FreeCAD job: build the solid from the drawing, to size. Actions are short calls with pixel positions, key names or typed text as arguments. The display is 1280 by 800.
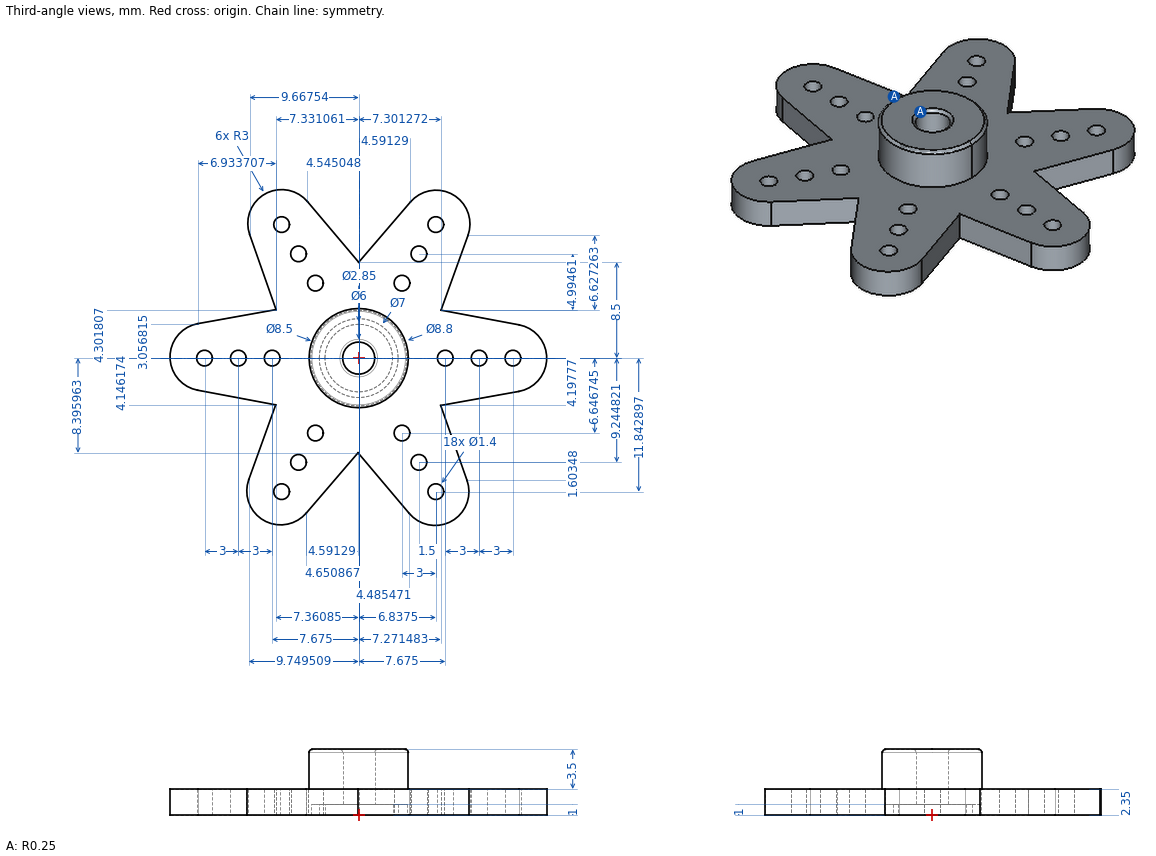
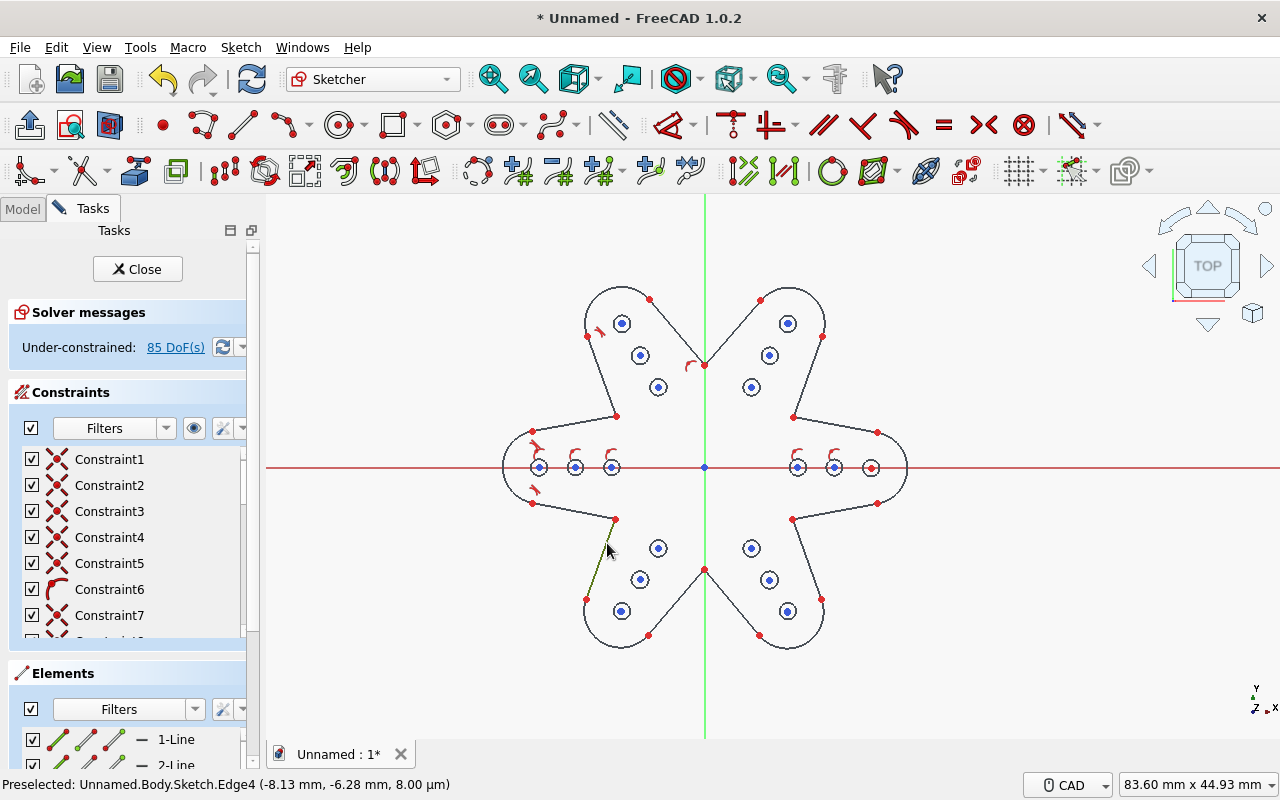
click(589, 628)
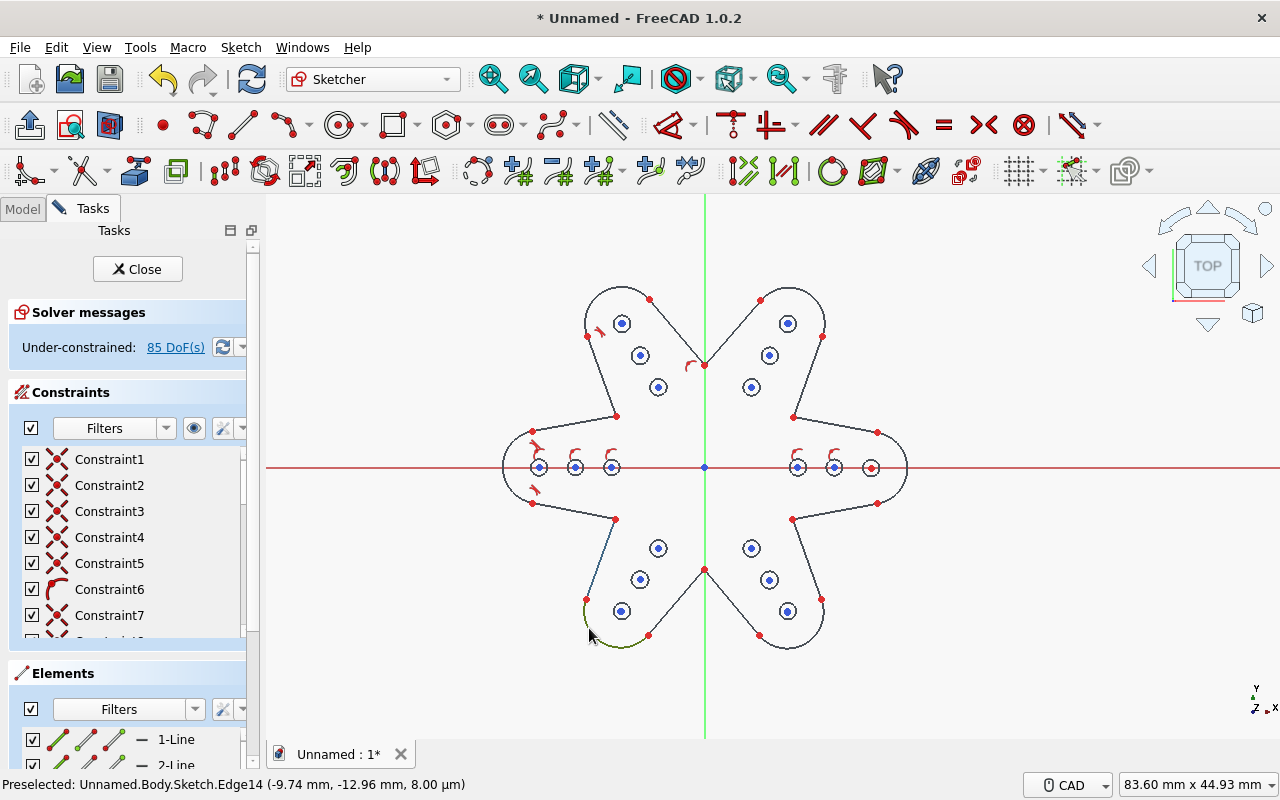
click(904, 126)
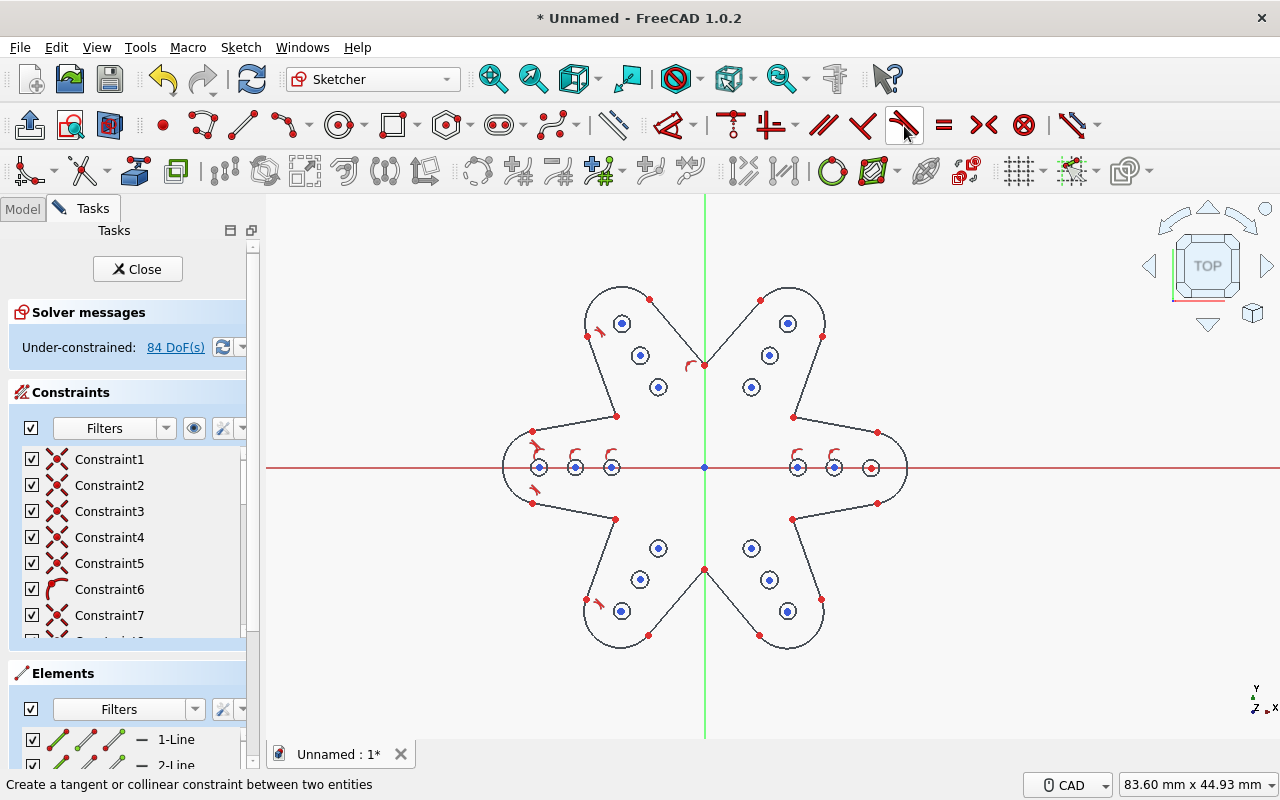
click(665, 615)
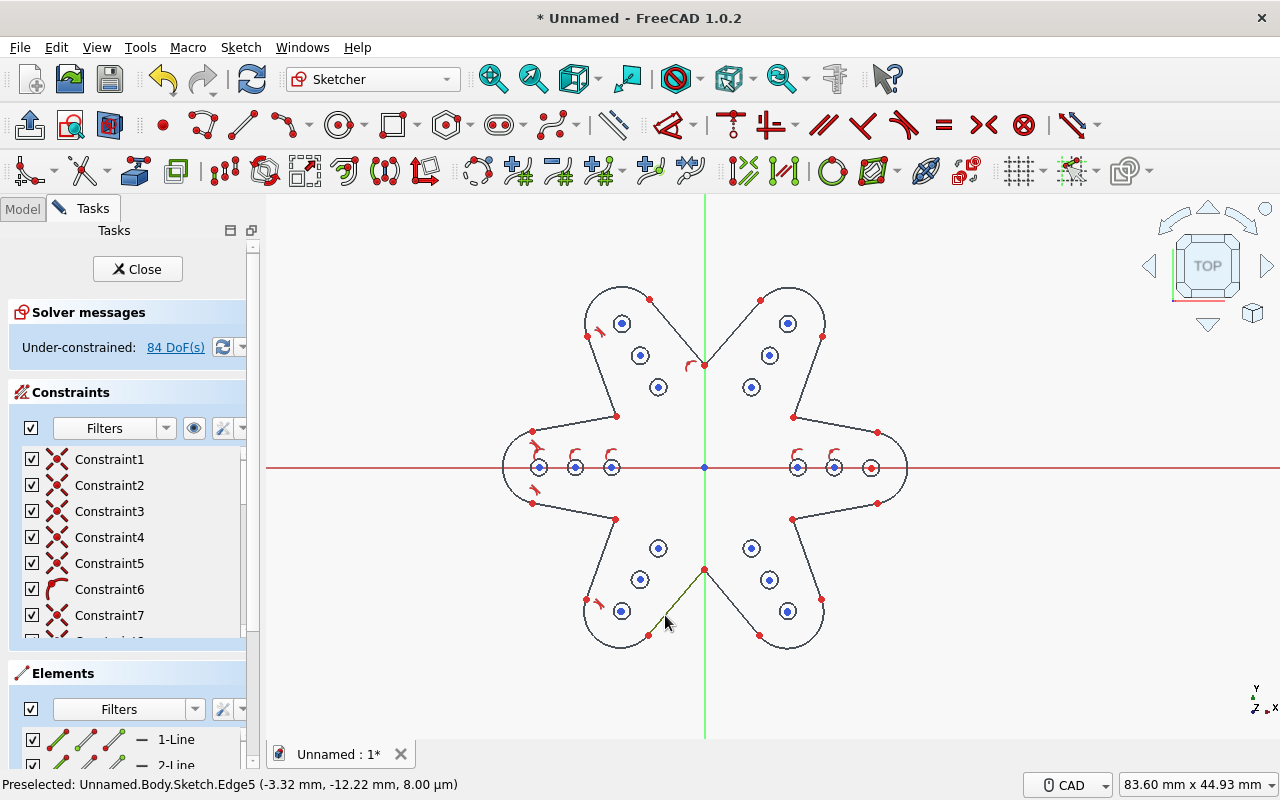
click(588, 628)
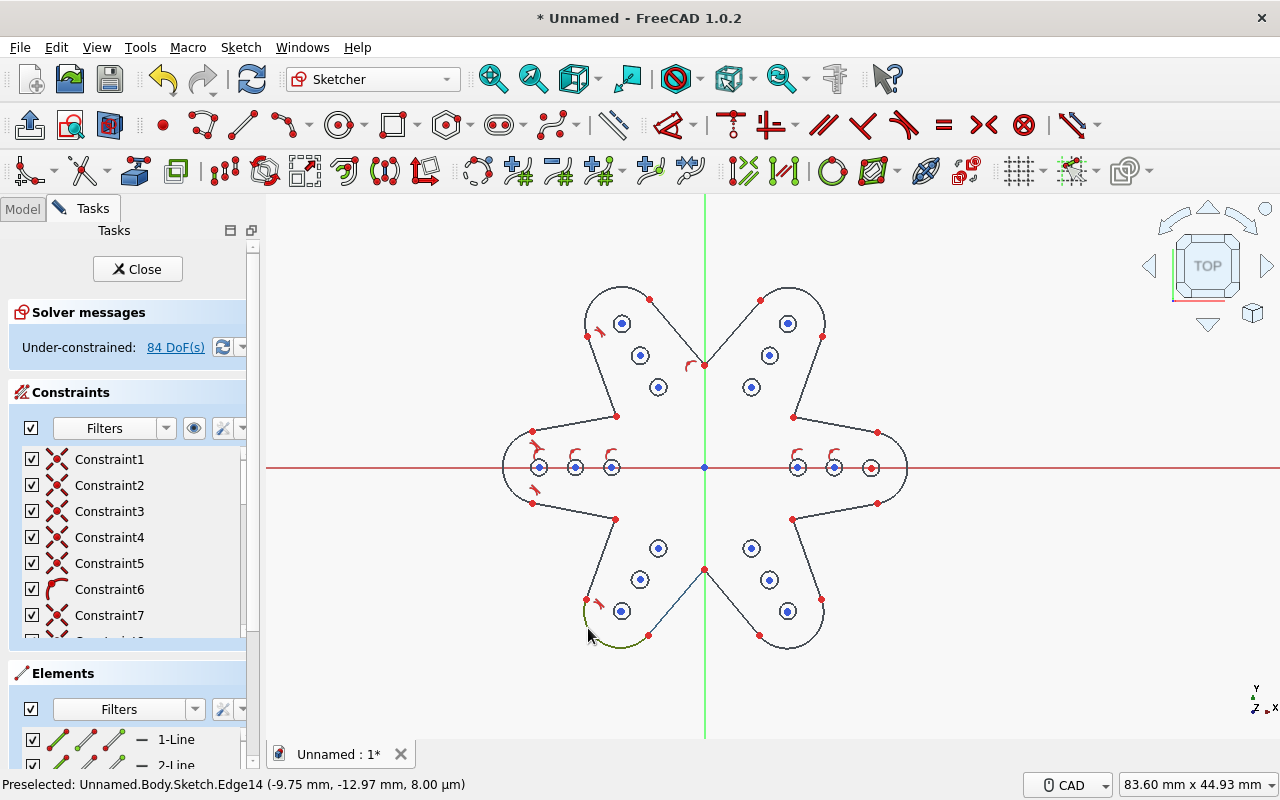
click(904, 126)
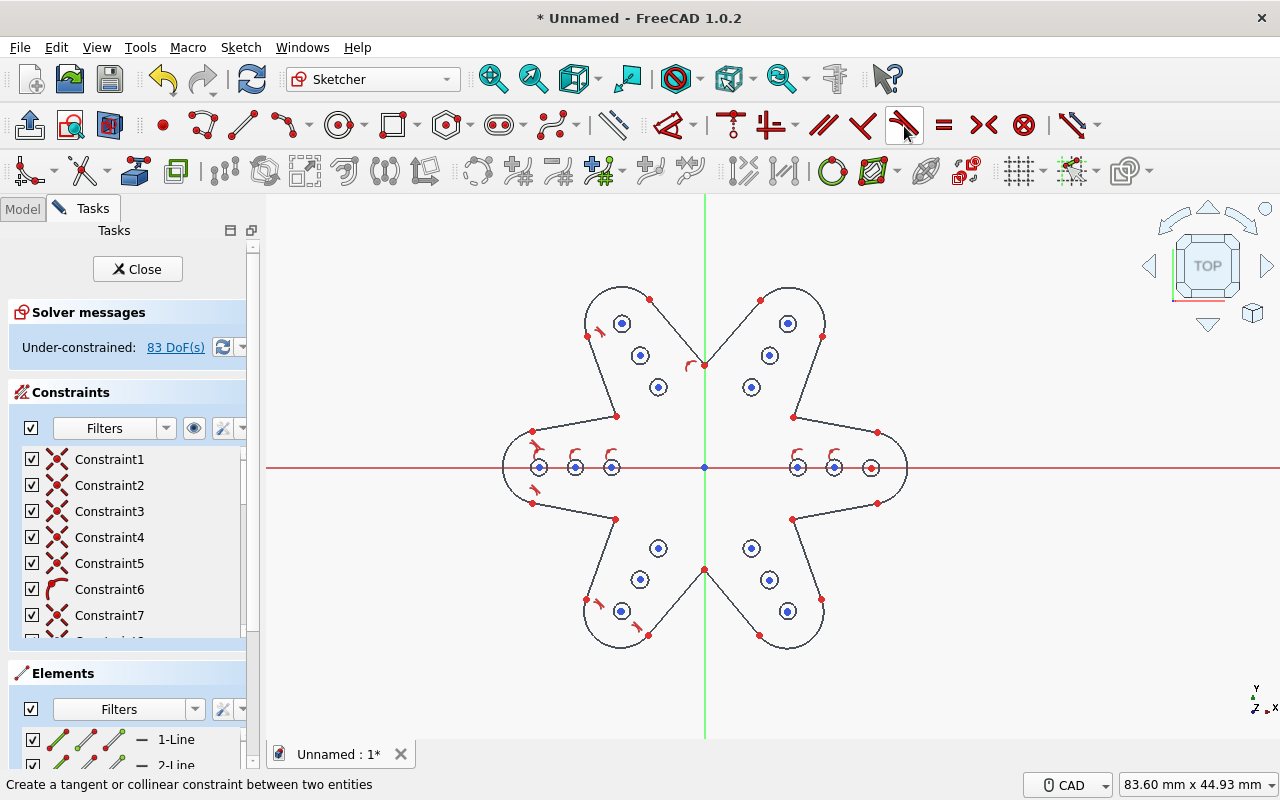
click(721, 589)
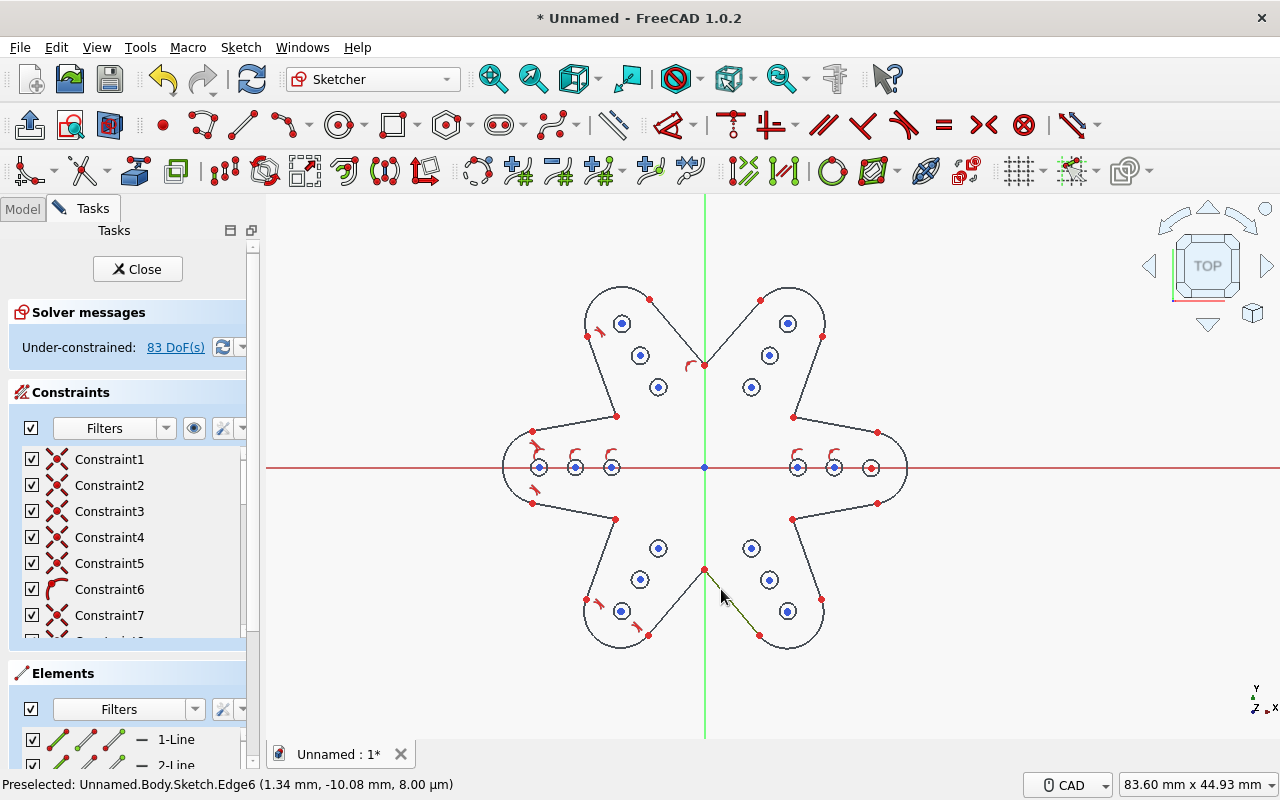
click(786, 649)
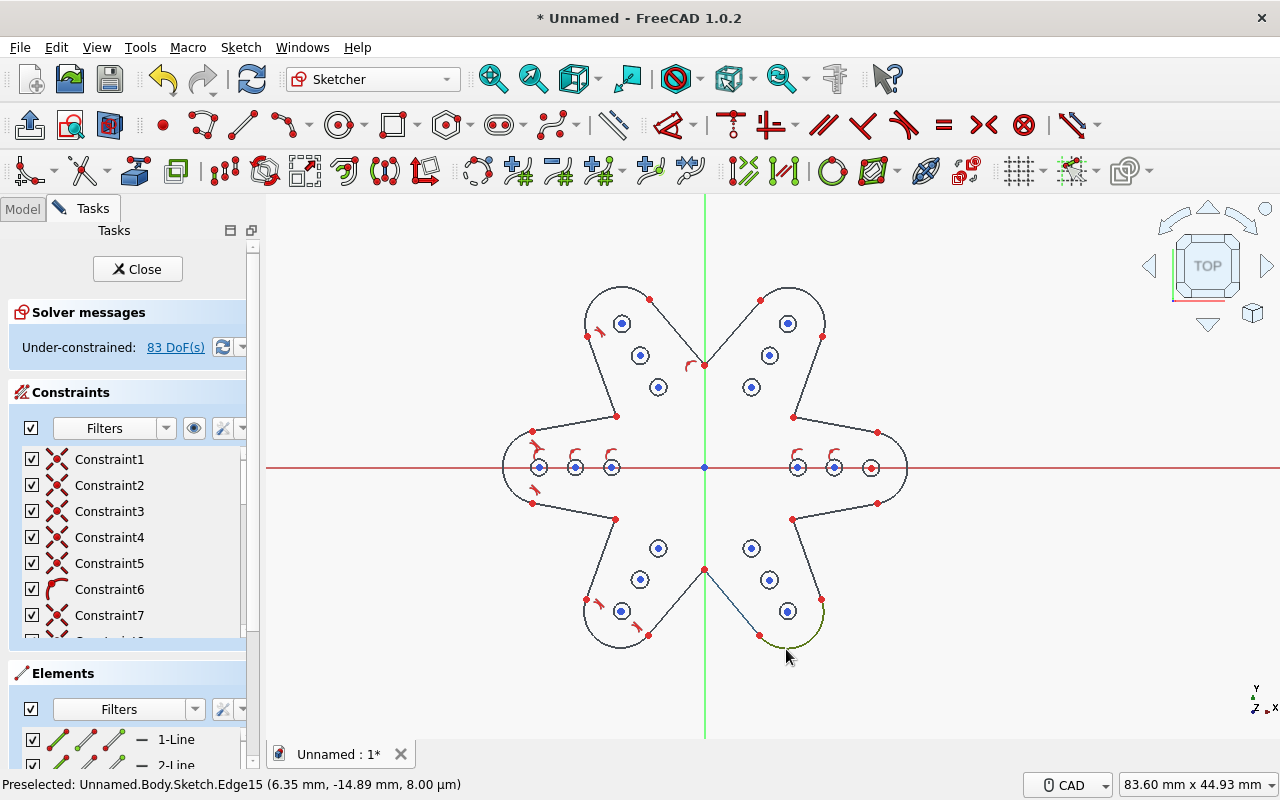
click(904, 126)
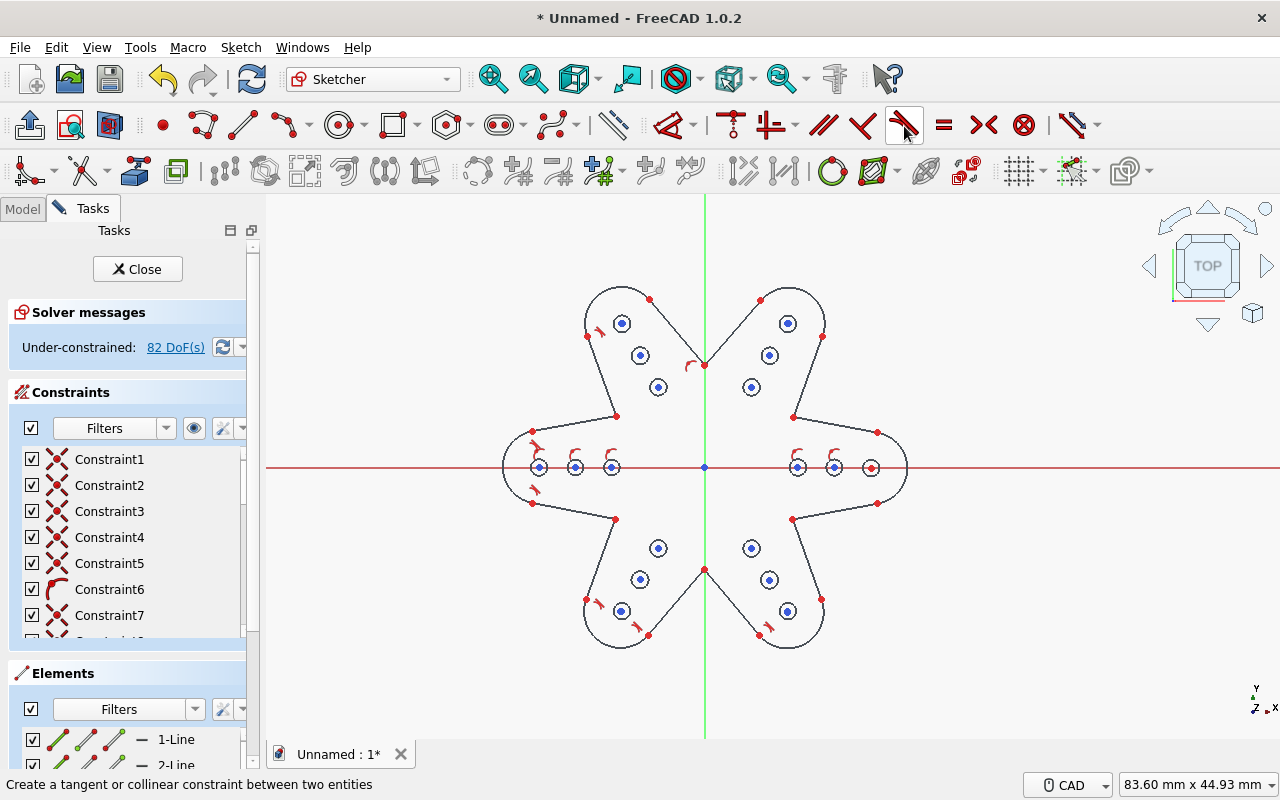
click(813, 576)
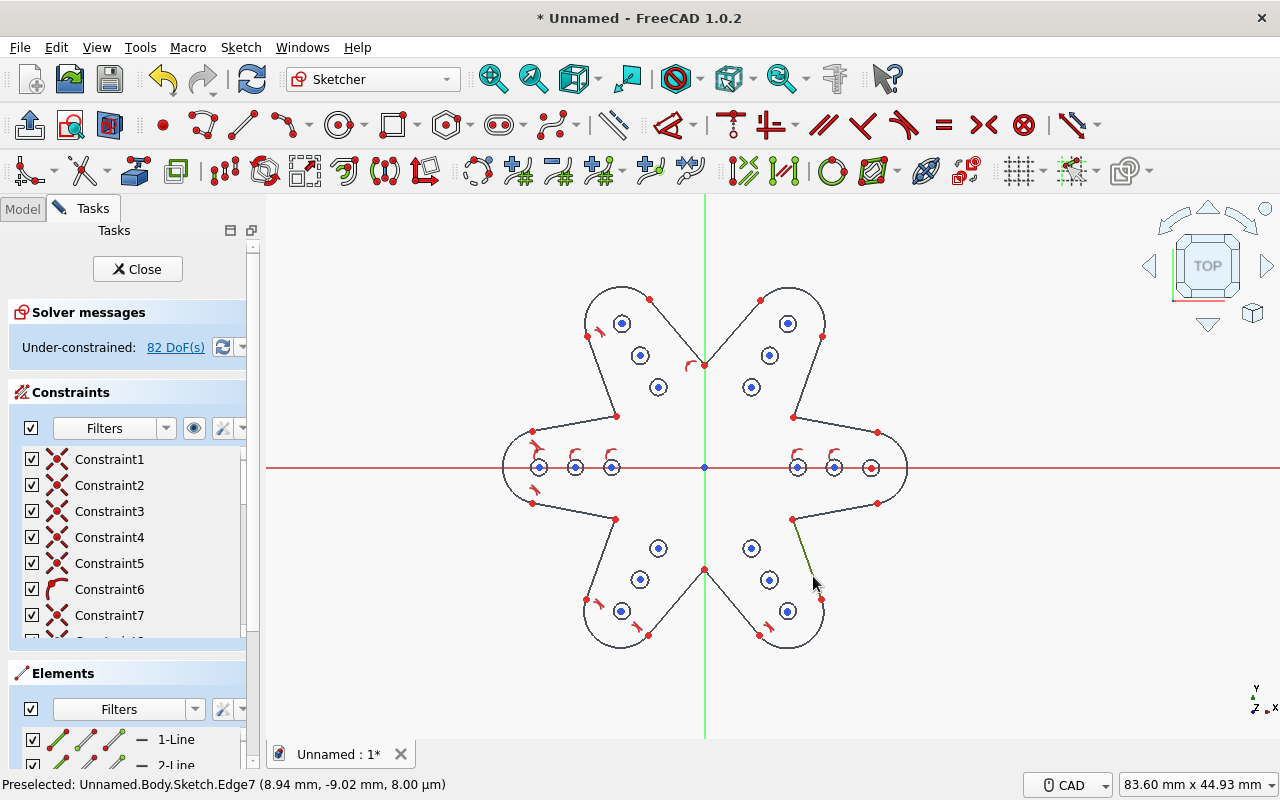
click(786, 648)